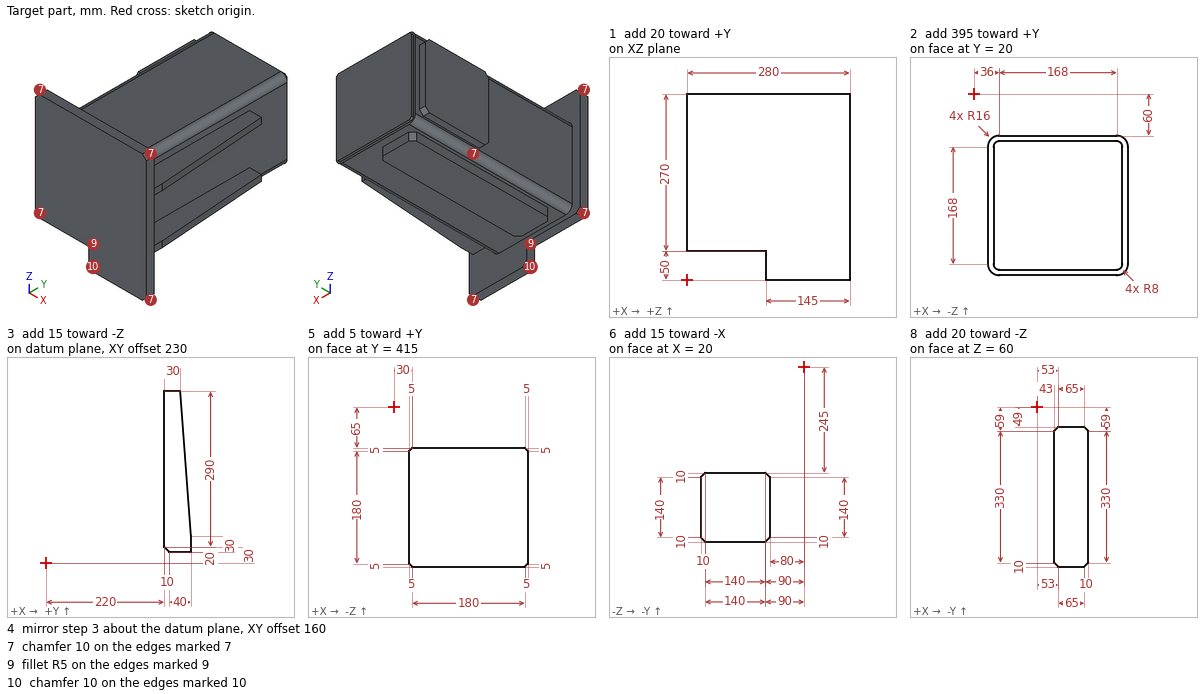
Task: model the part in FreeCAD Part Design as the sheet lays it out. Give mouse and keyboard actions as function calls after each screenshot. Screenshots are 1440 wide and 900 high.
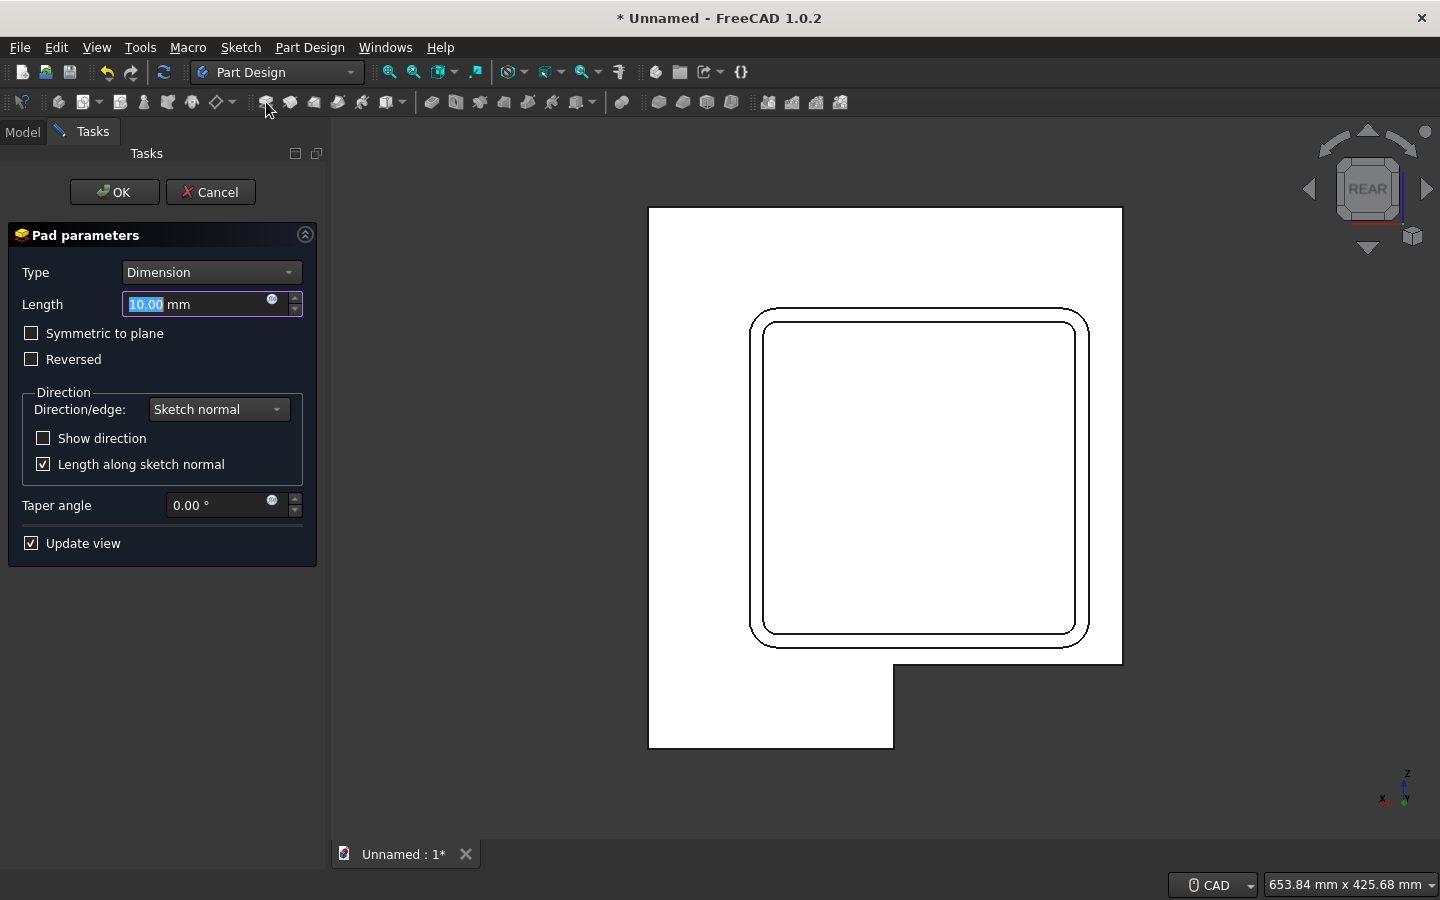
text(395)
key(Tab)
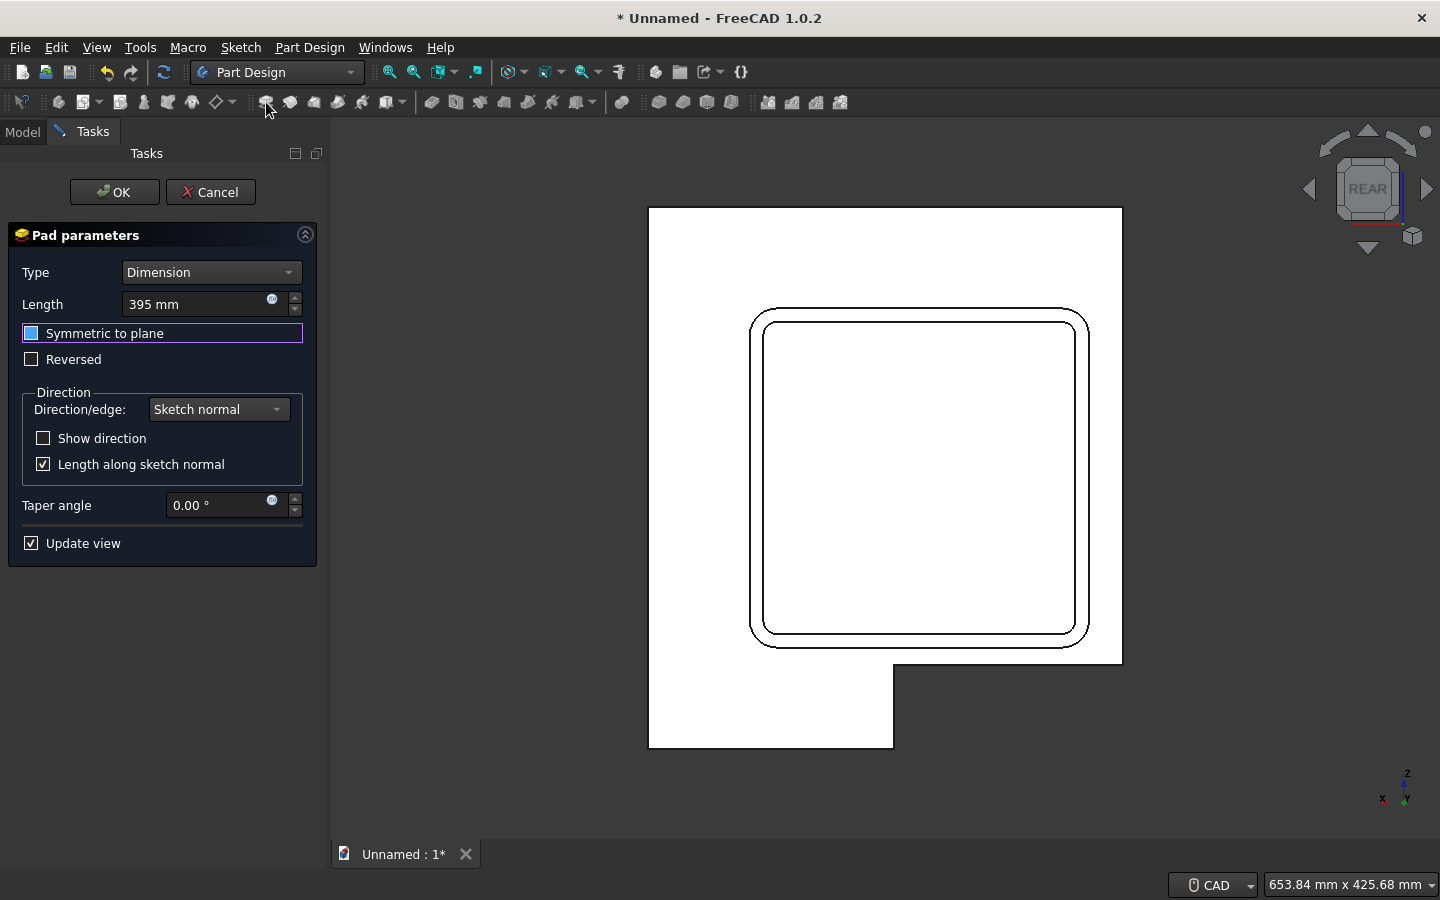
click(115, 192)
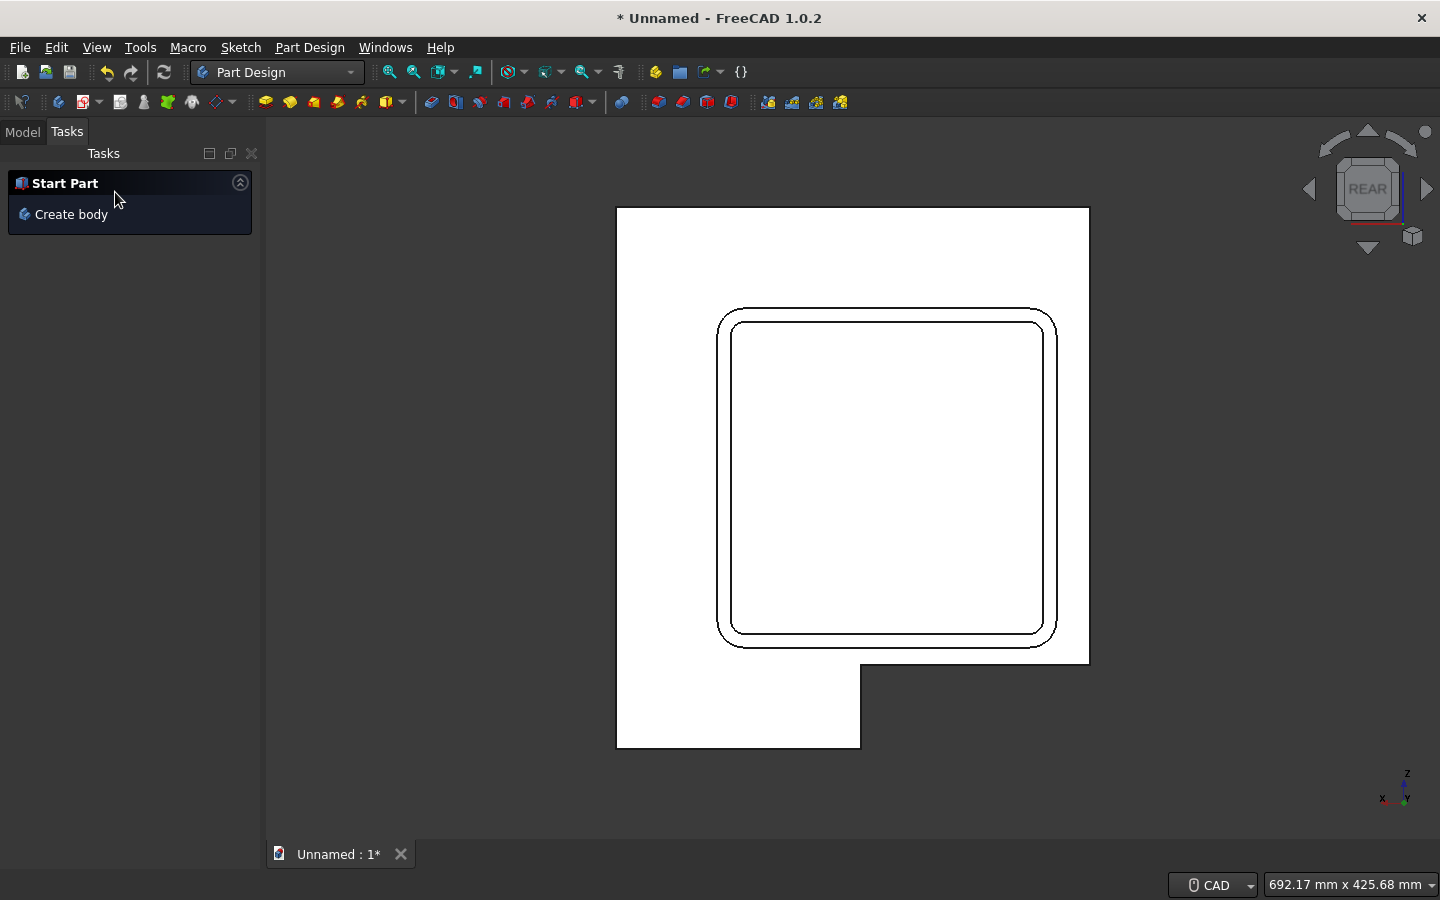
click(23, 131)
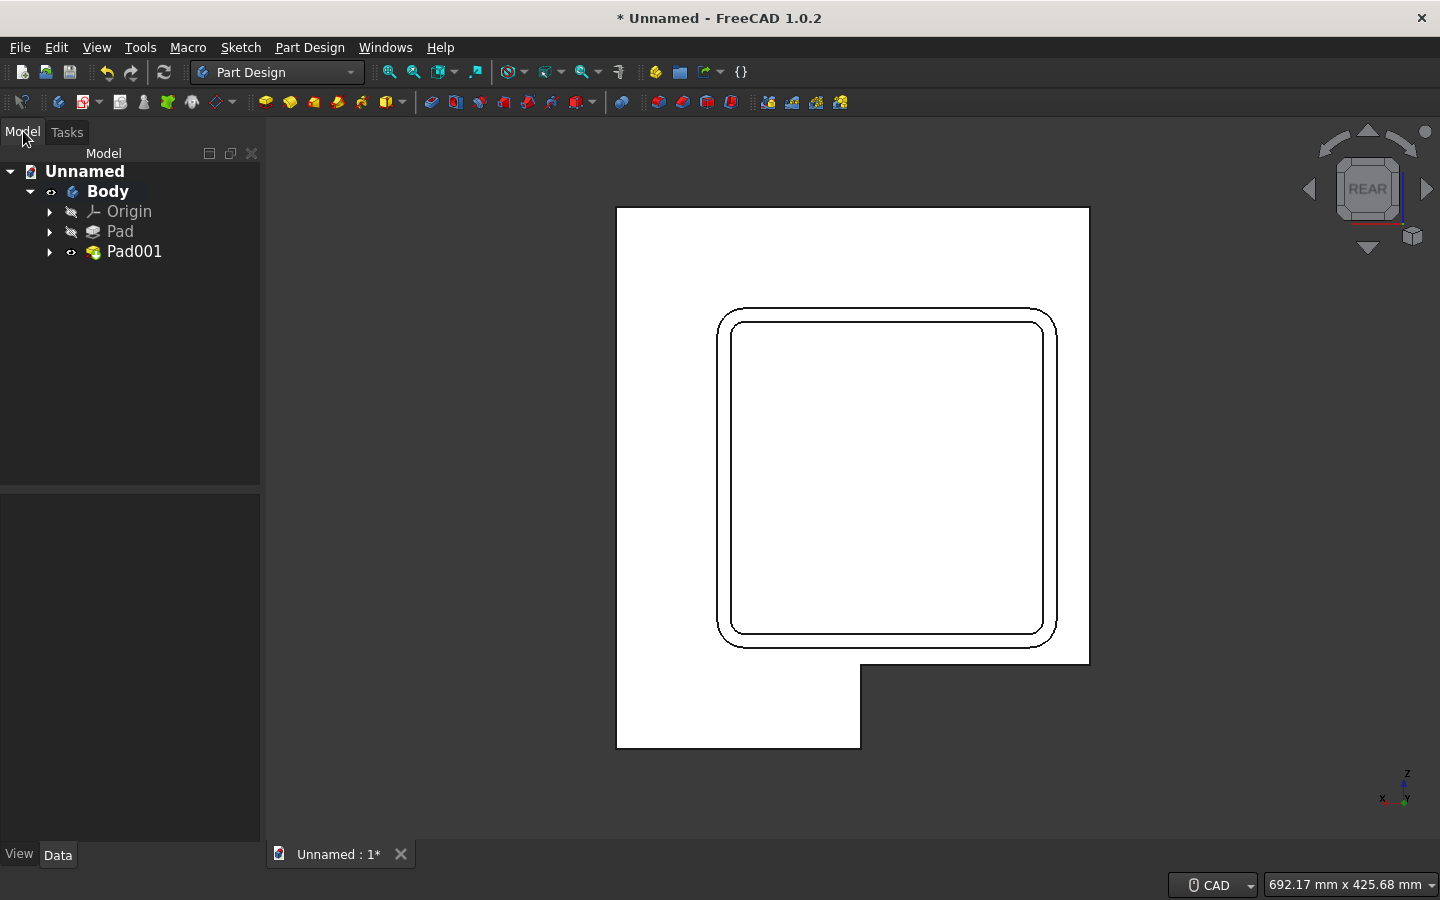
click(50, 212)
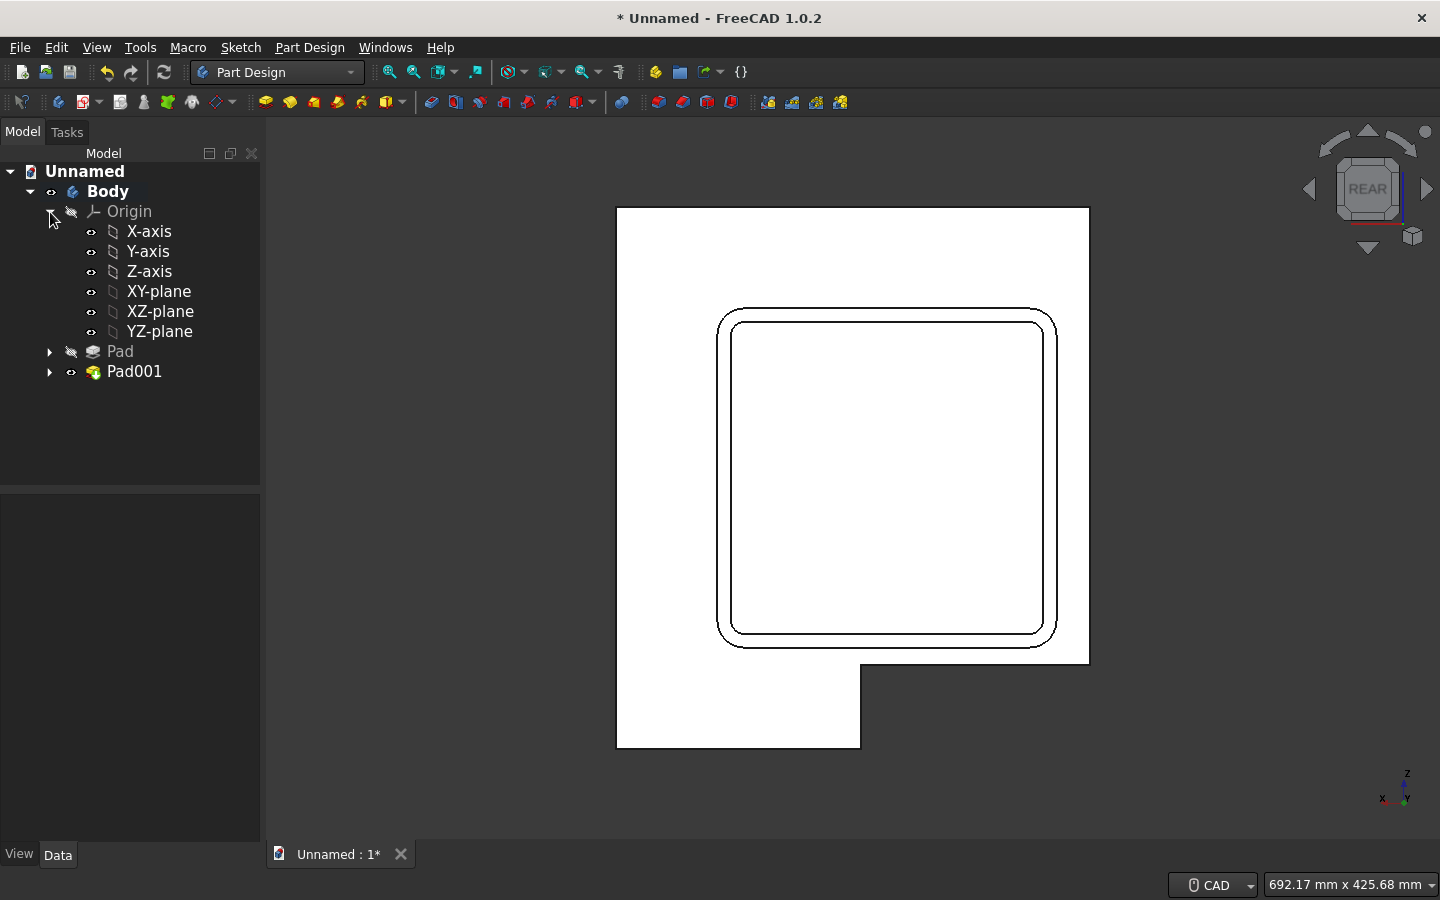
click(136, 292)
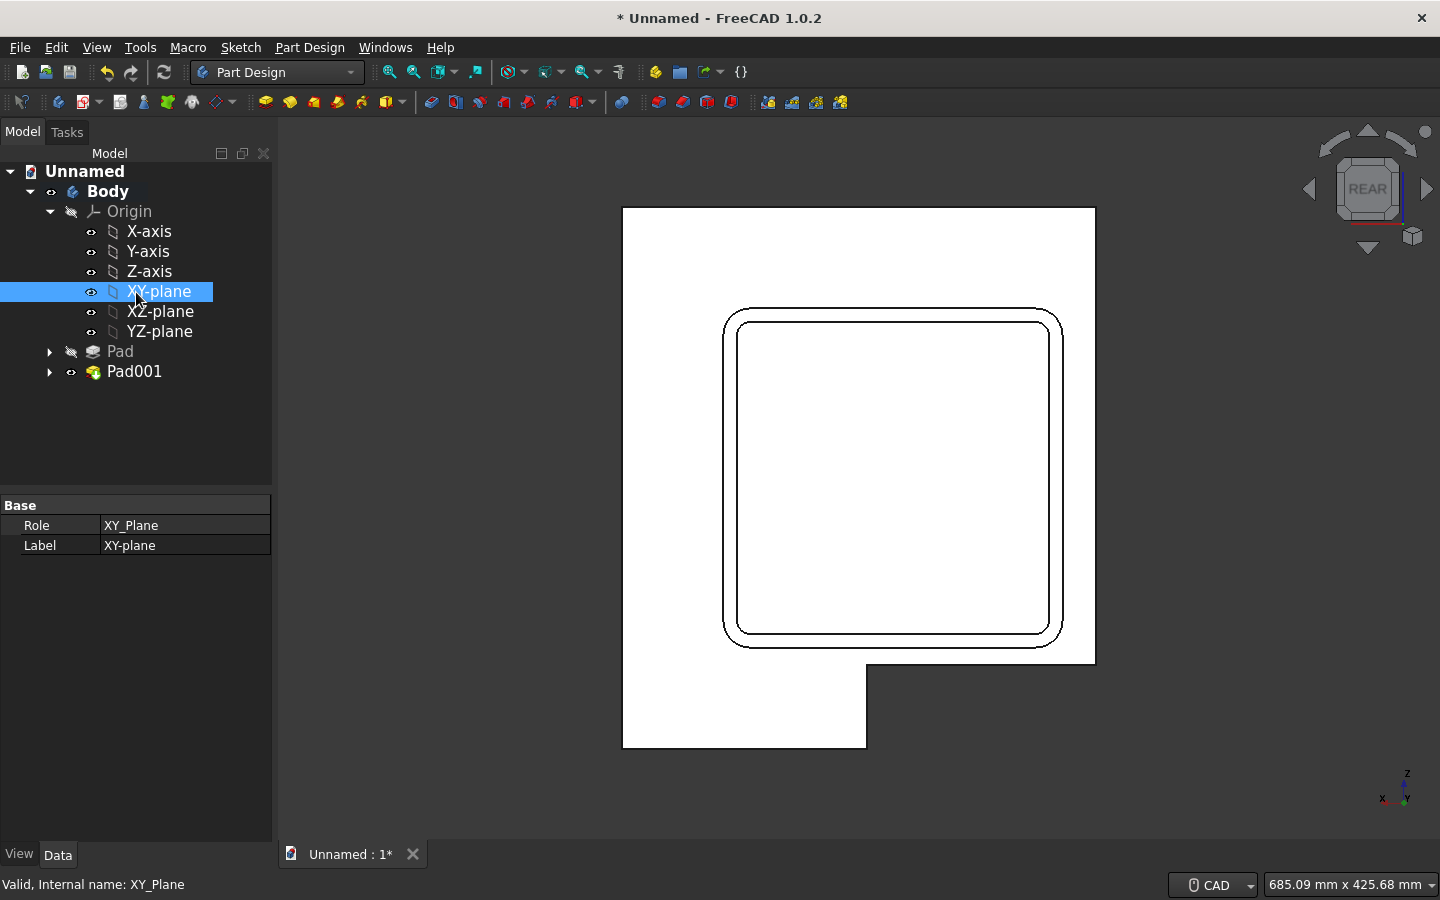
click(216, 102)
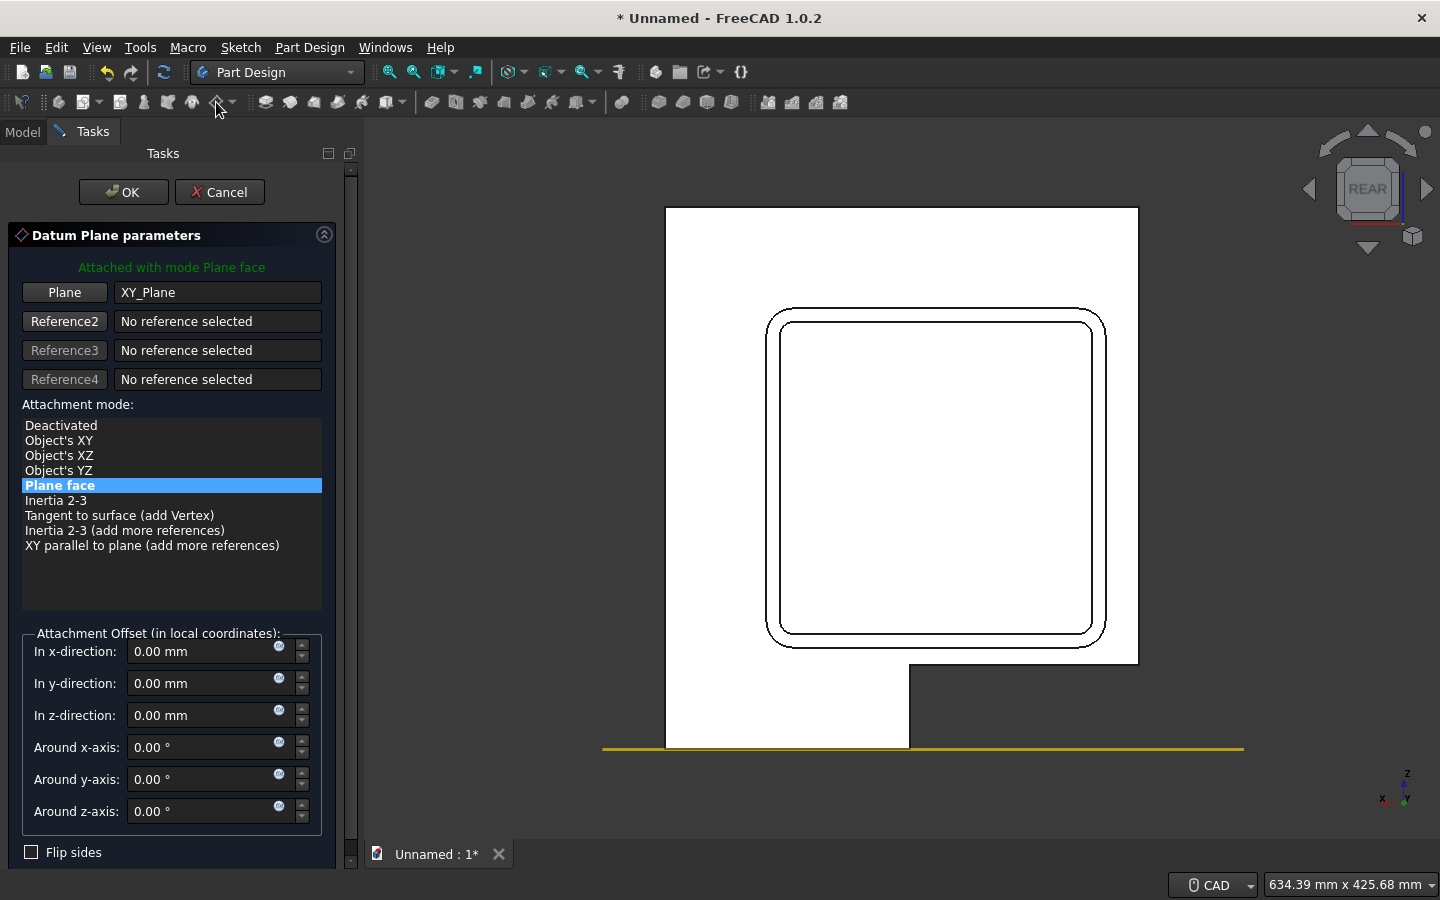
triple_click(210, 715)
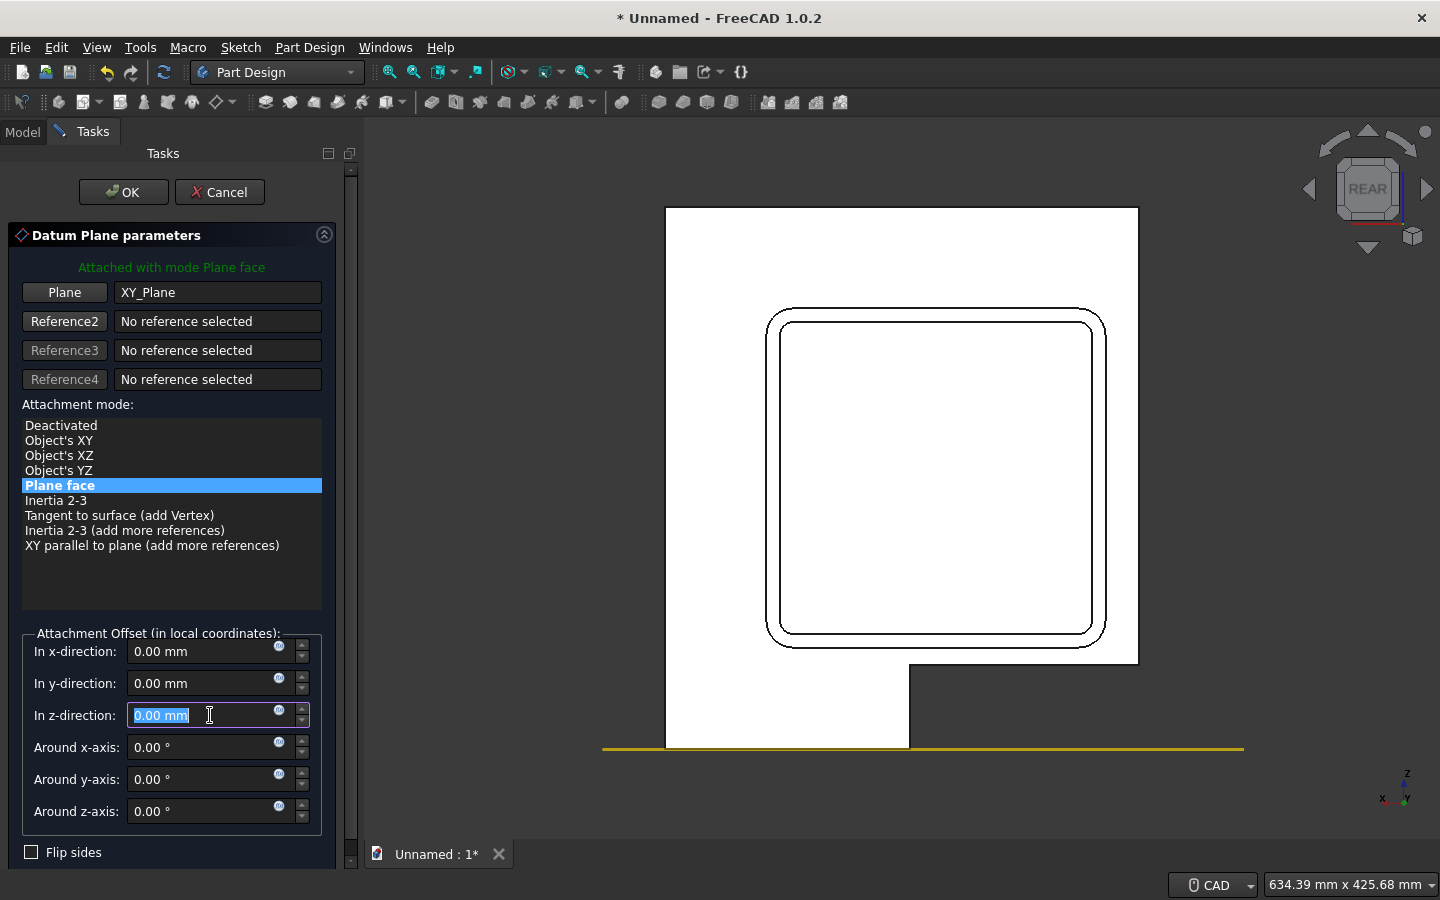
text(230)
key(Tab)